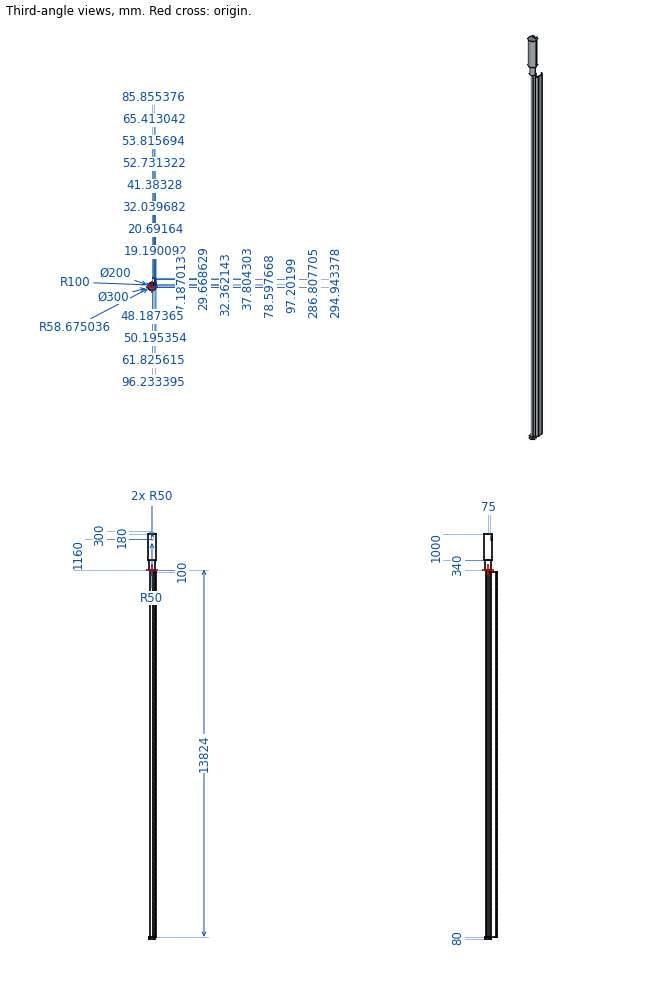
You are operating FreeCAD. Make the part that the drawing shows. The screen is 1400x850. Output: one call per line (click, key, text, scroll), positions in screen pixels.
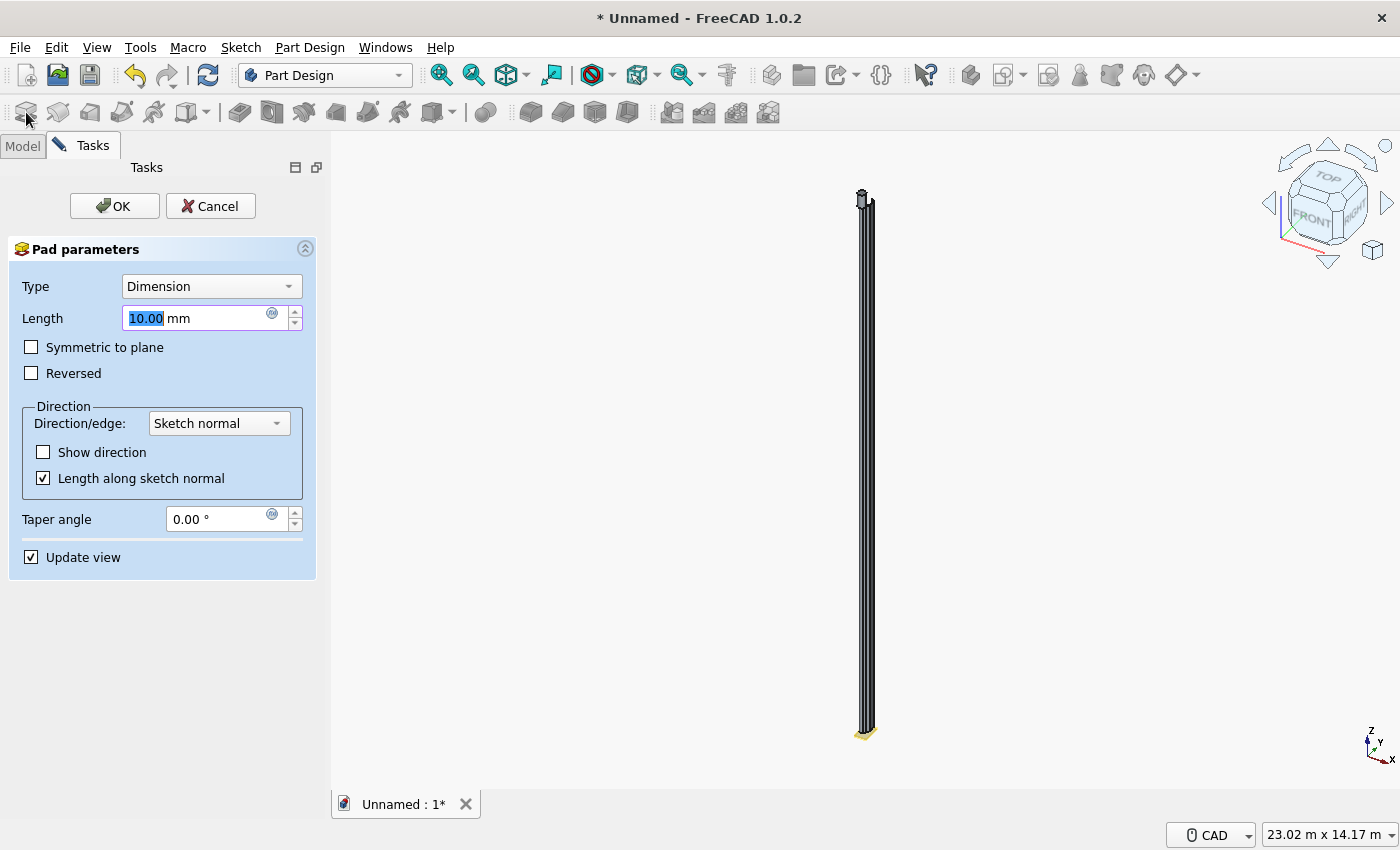
text(80)
key(Tab)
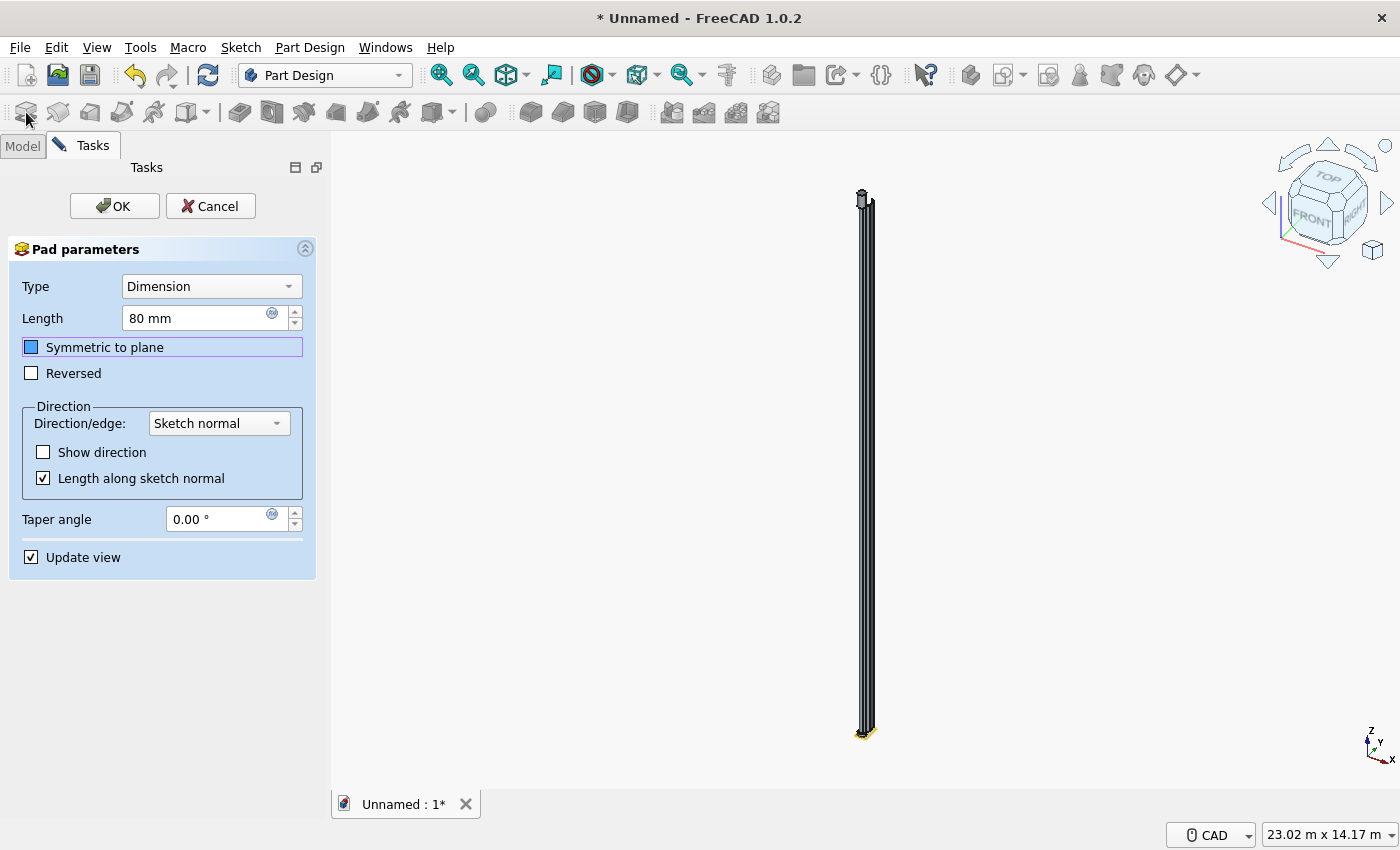
click(115, 206)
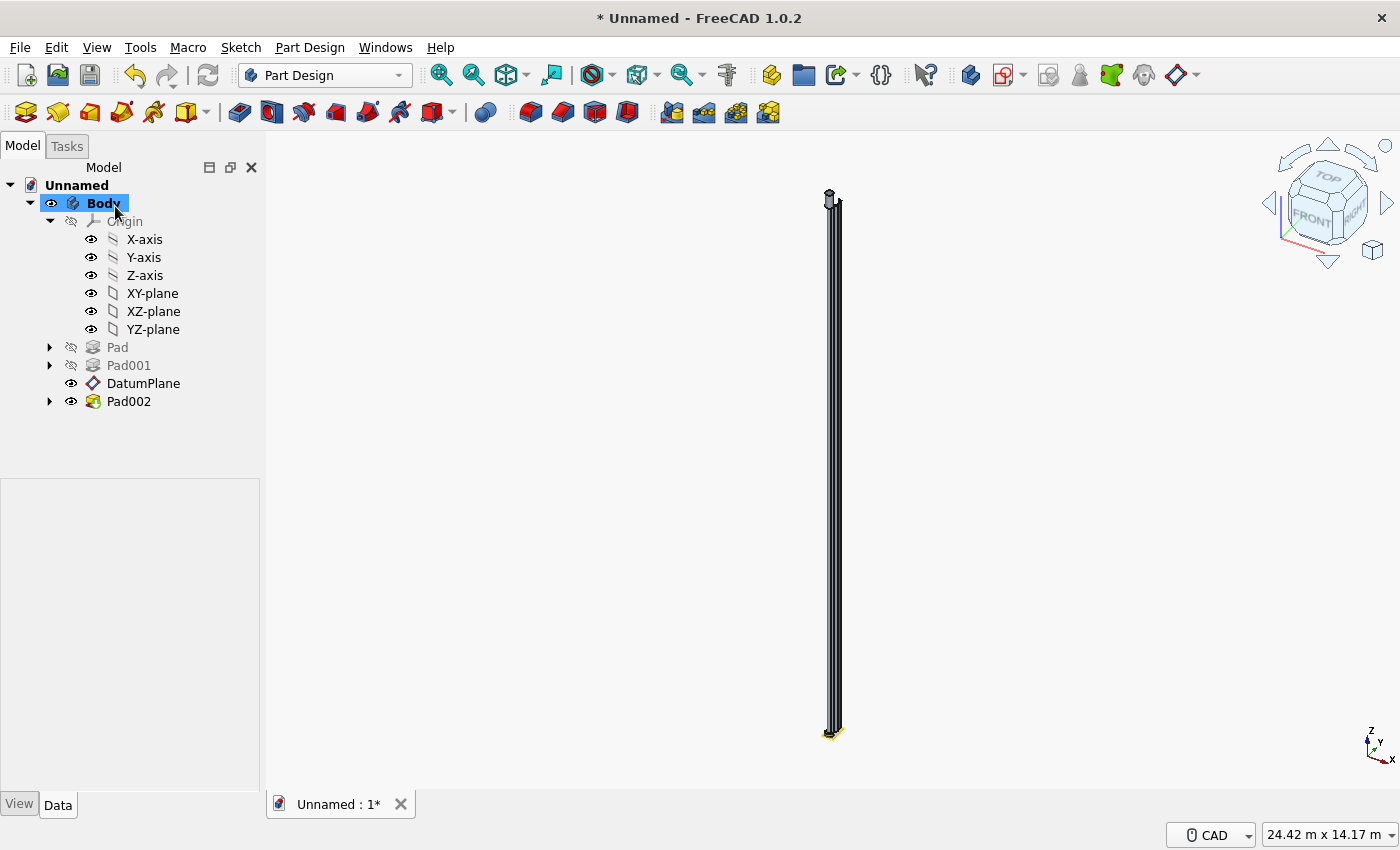
click(116, 383)
key(space)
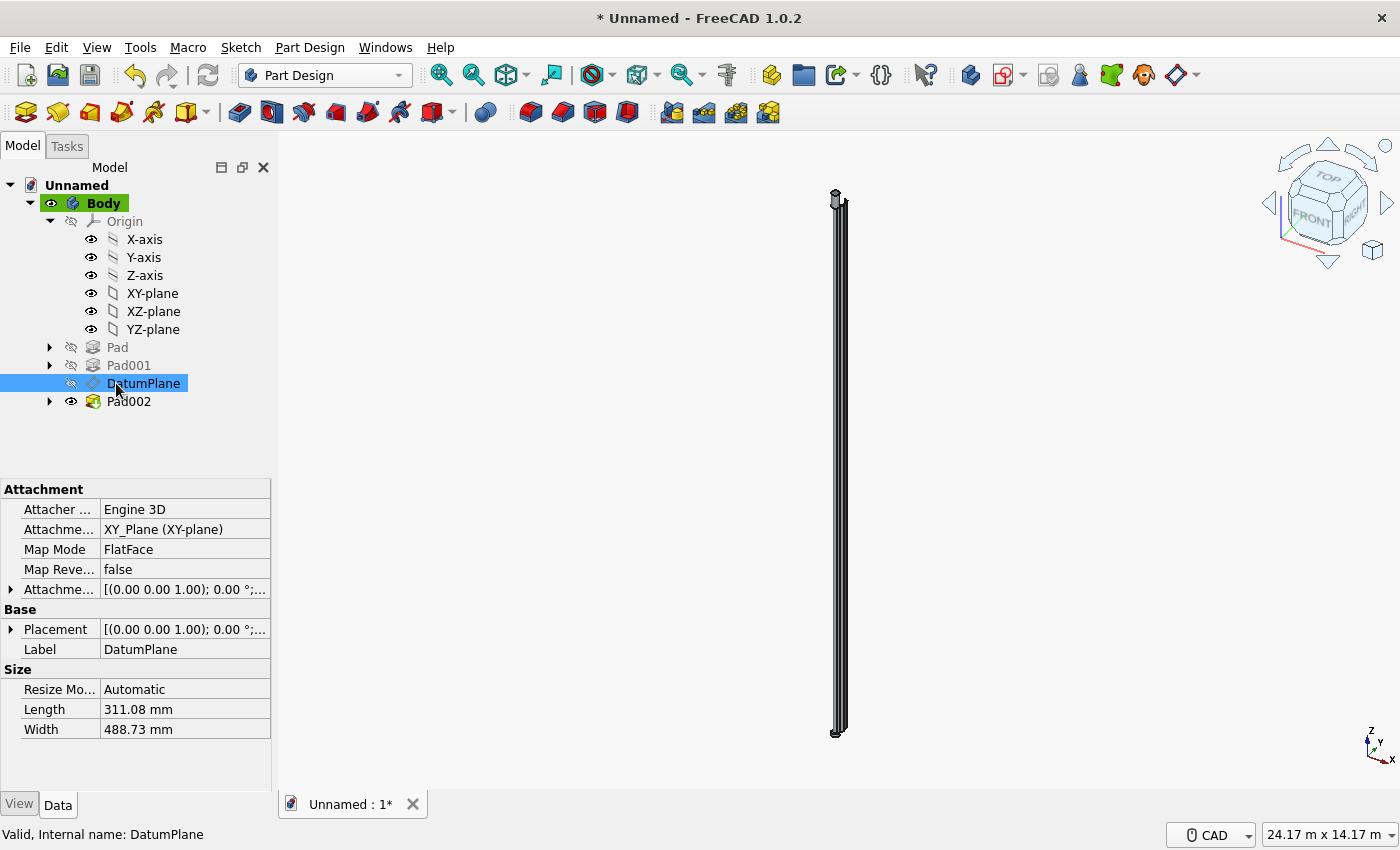
click(136, 293)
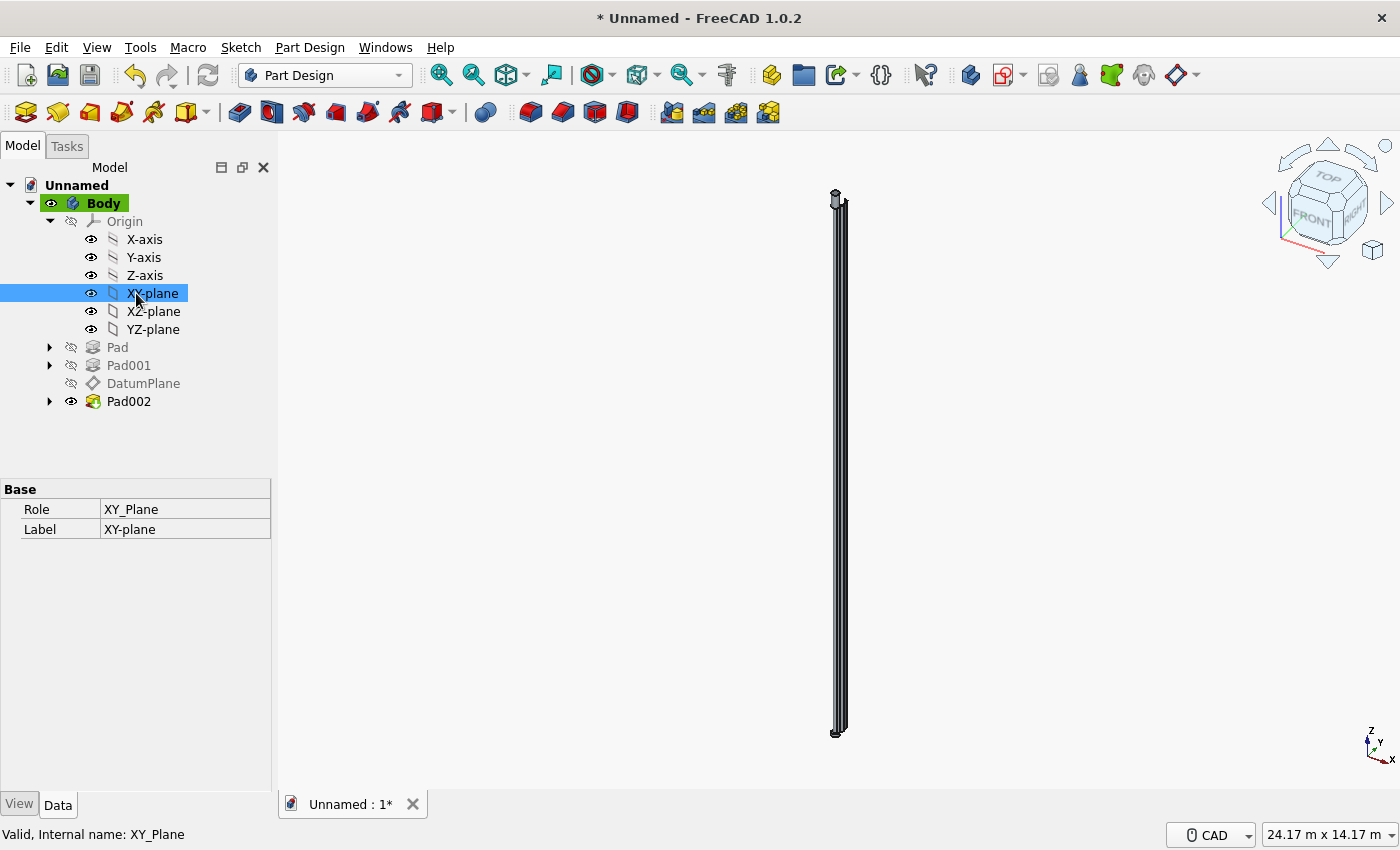
click(1176, 76)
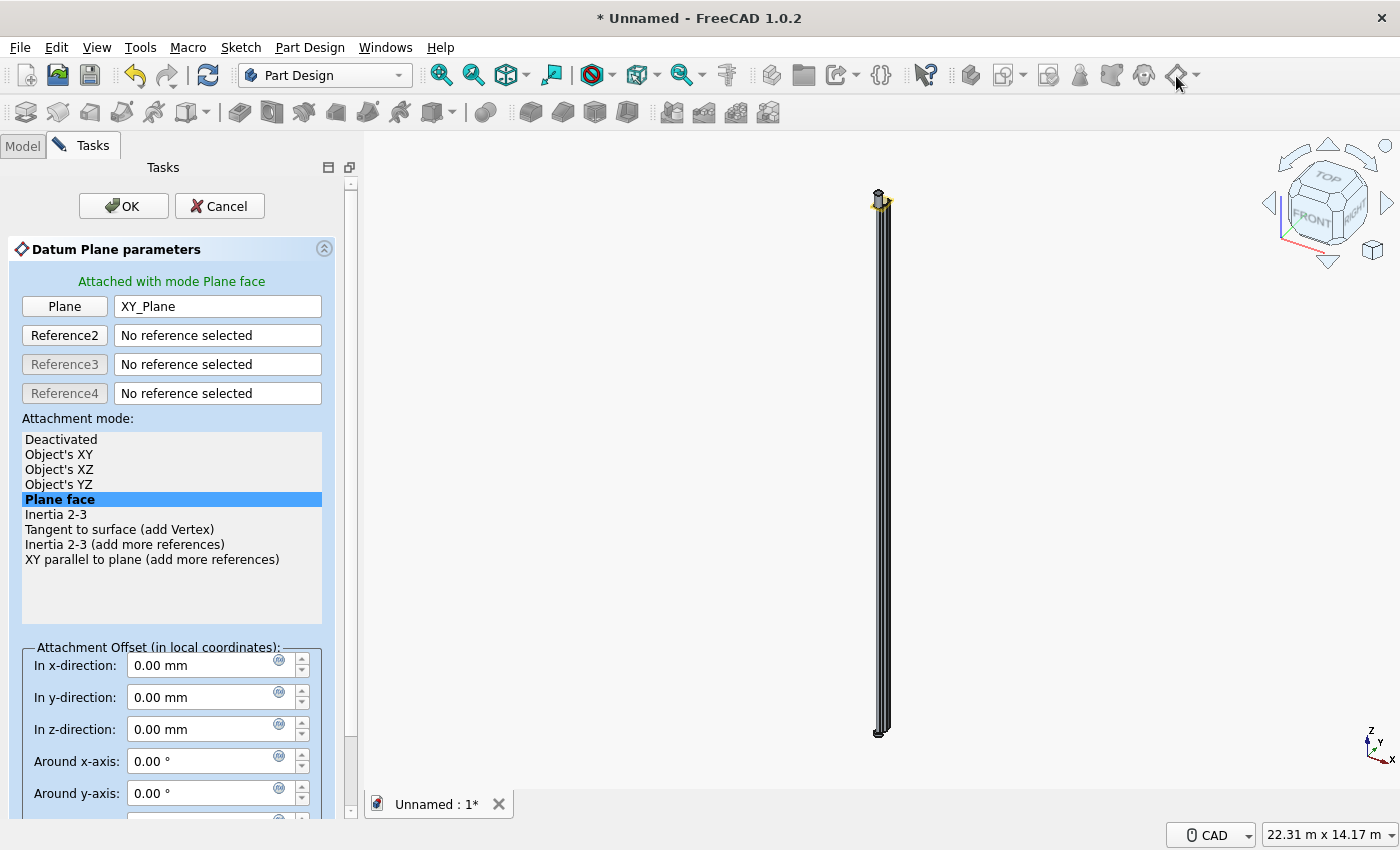
triple_click(210, 729)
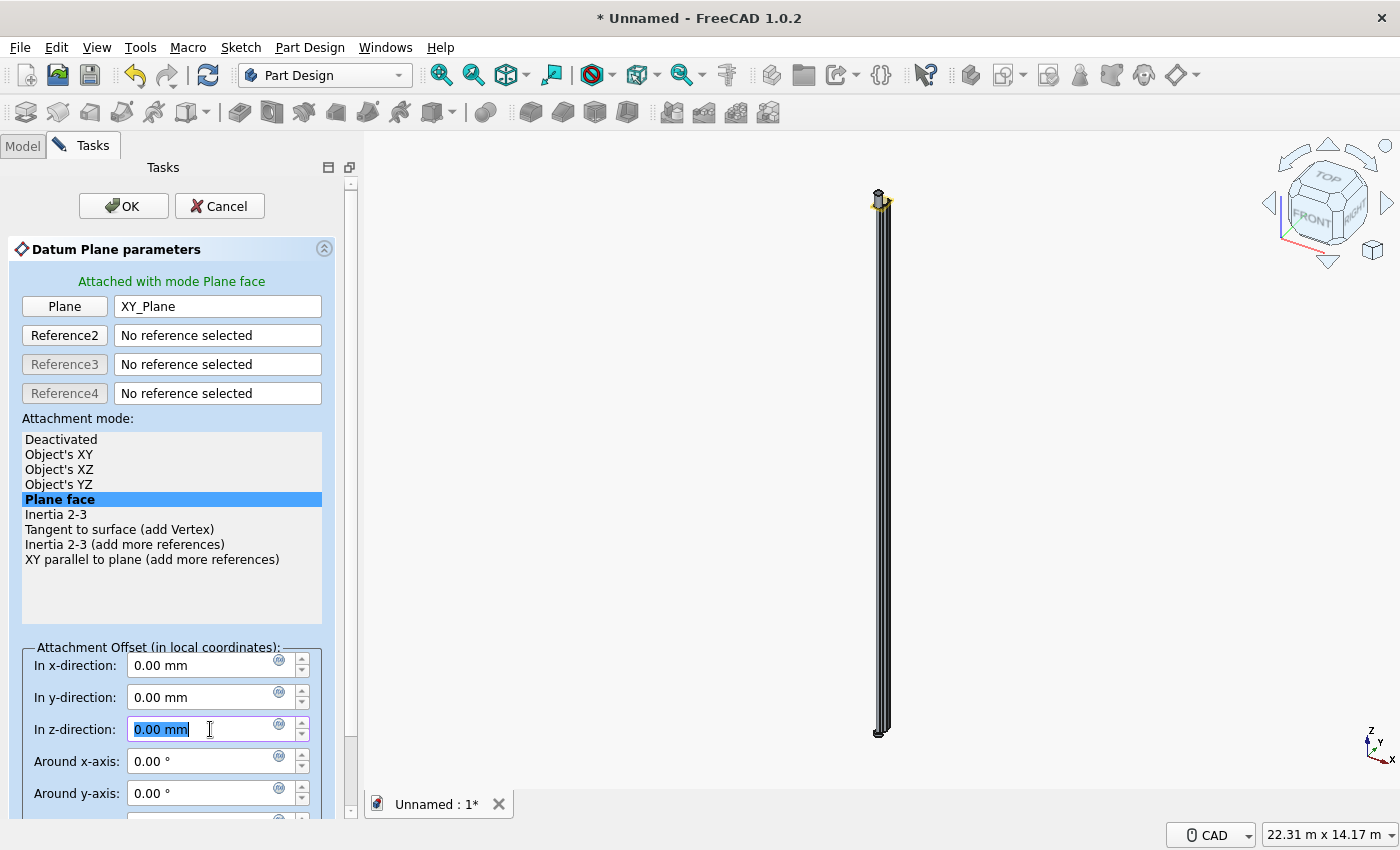
text(-100)
key(Tab)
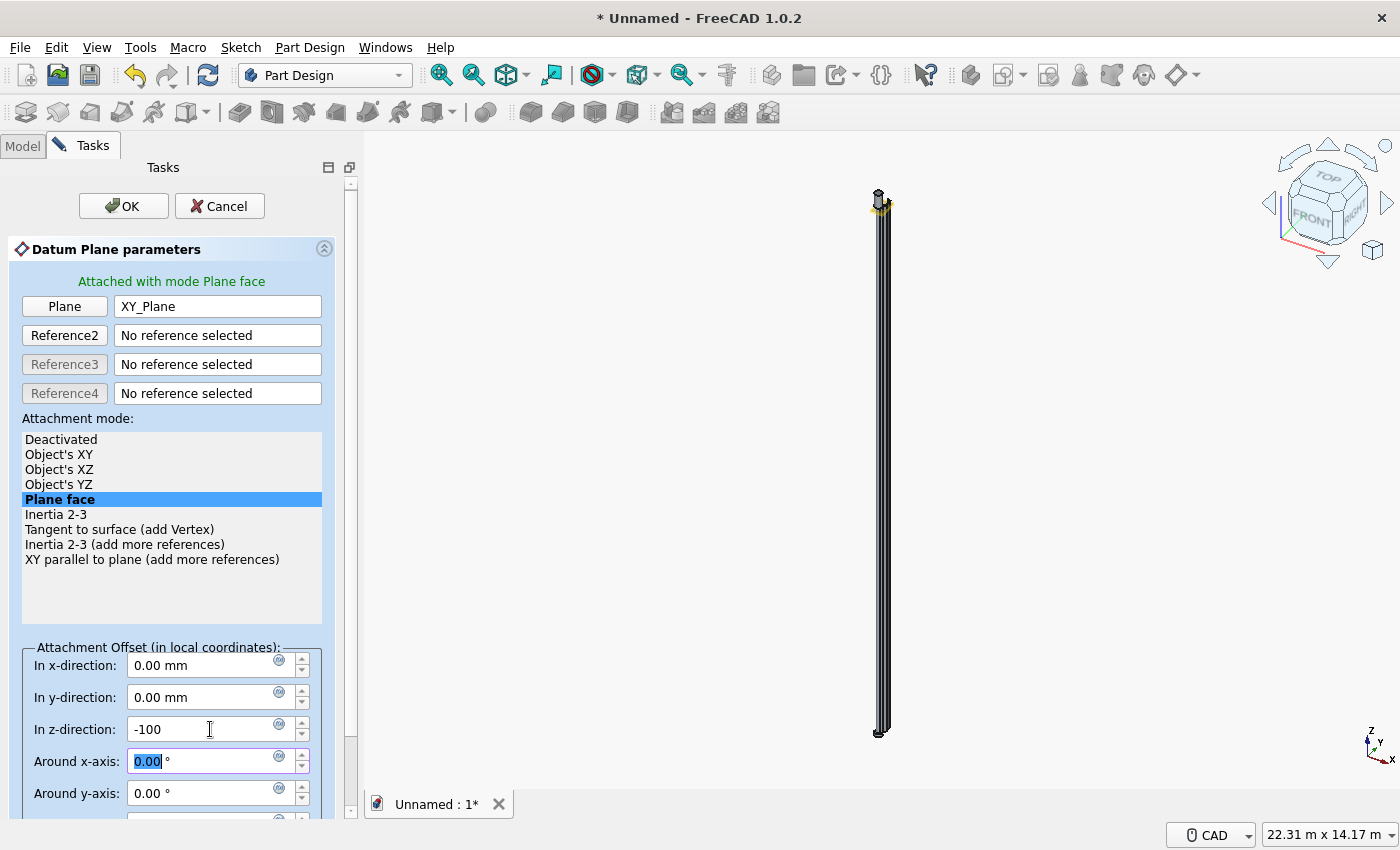
click(124, 206)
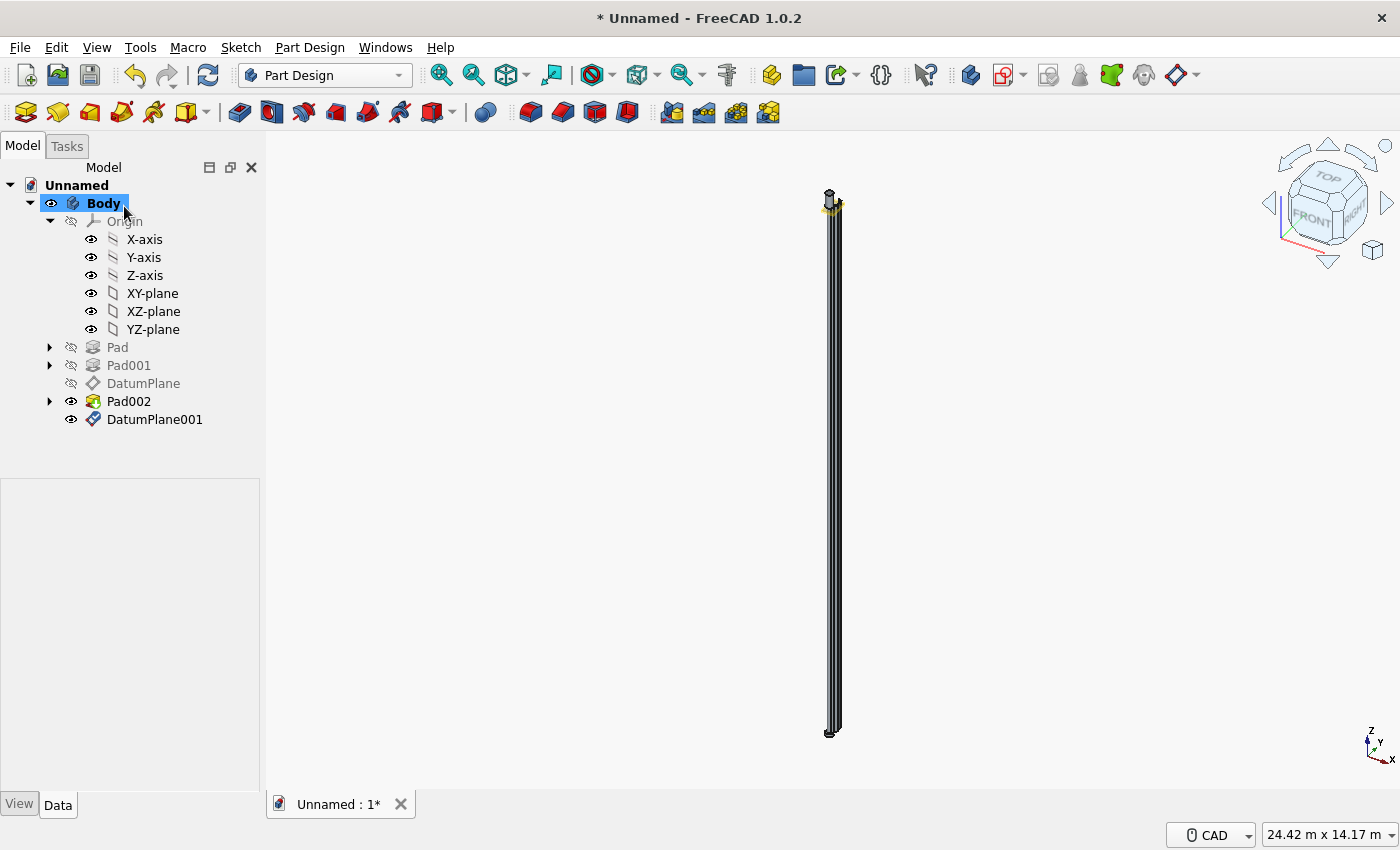
click(116, 419)